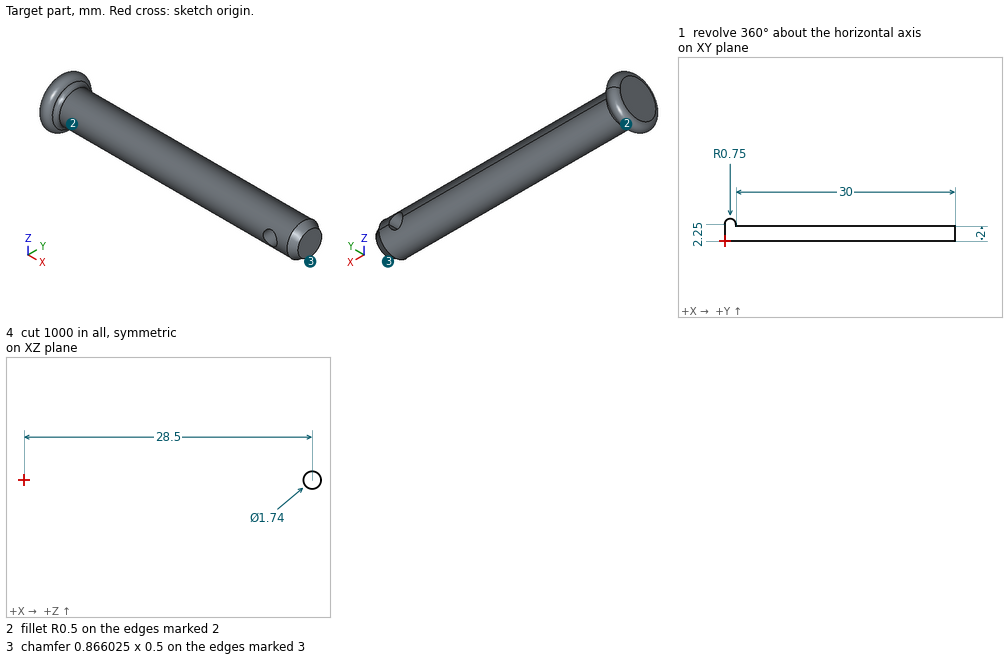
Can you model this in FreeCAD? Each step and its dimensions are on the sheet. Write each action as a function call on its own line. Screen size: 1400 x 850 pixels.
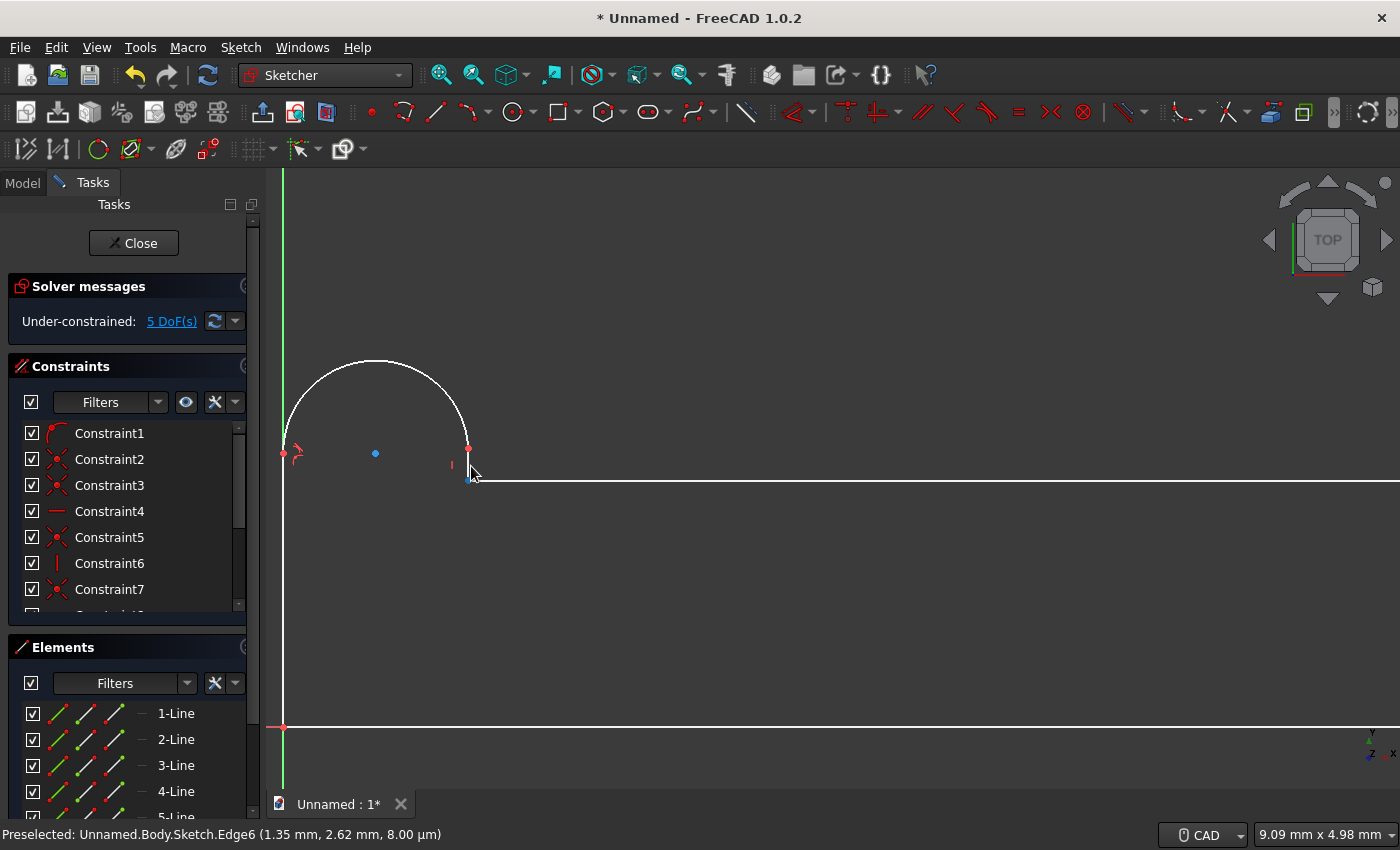
click(468, 465)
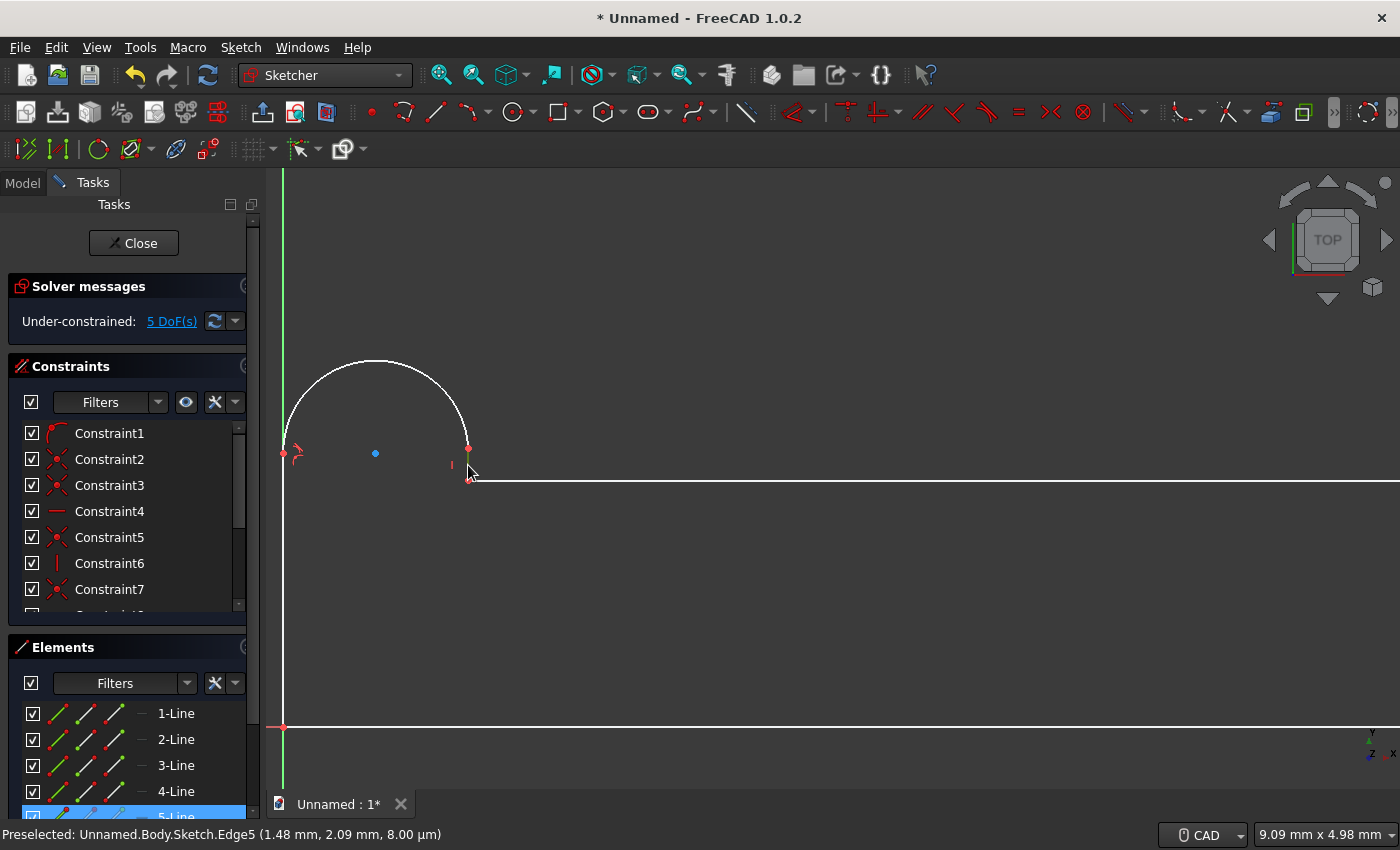
scroll(471, 466, down, 9)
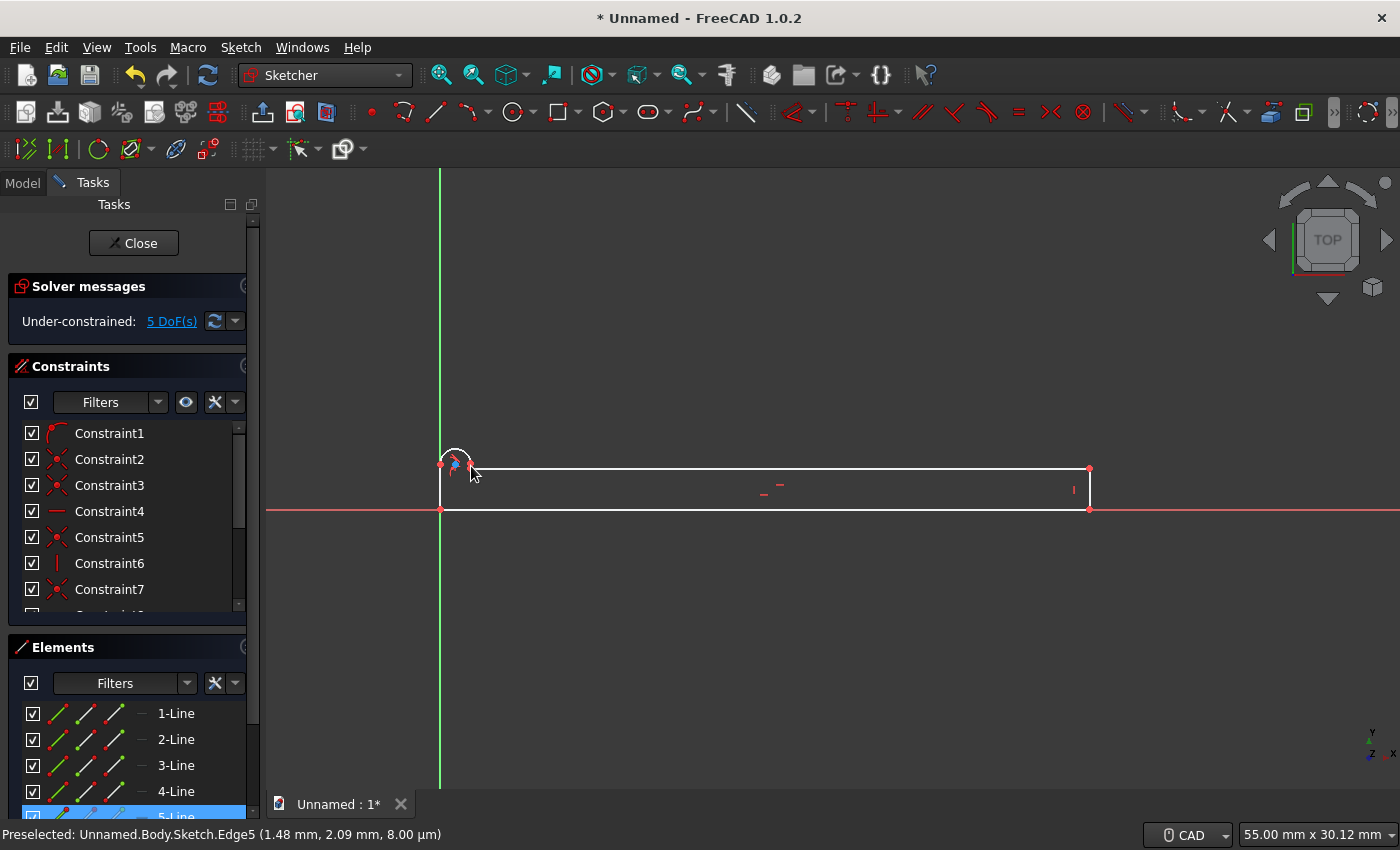
click(464, 452)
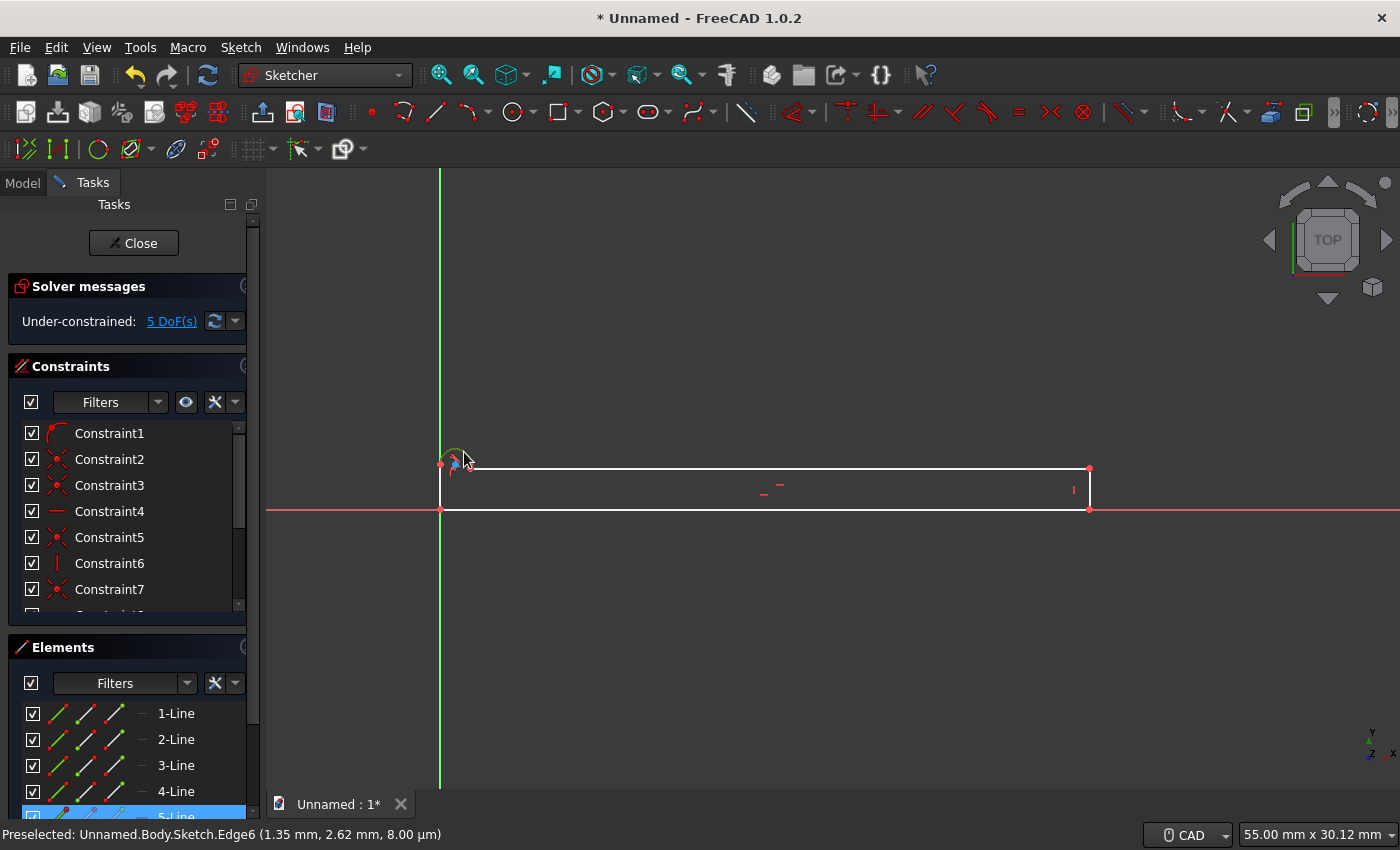
click(988, 112)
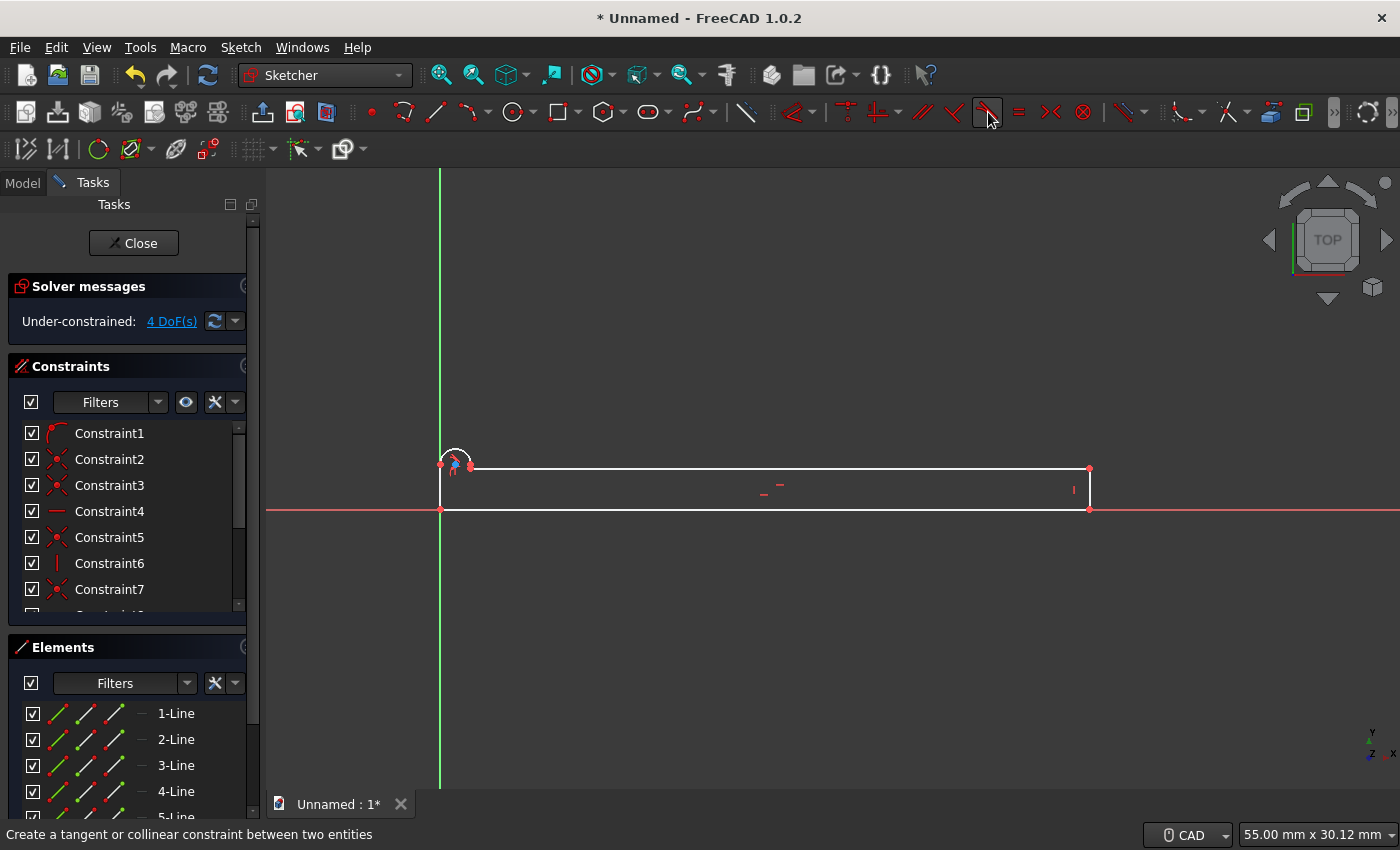
key(d)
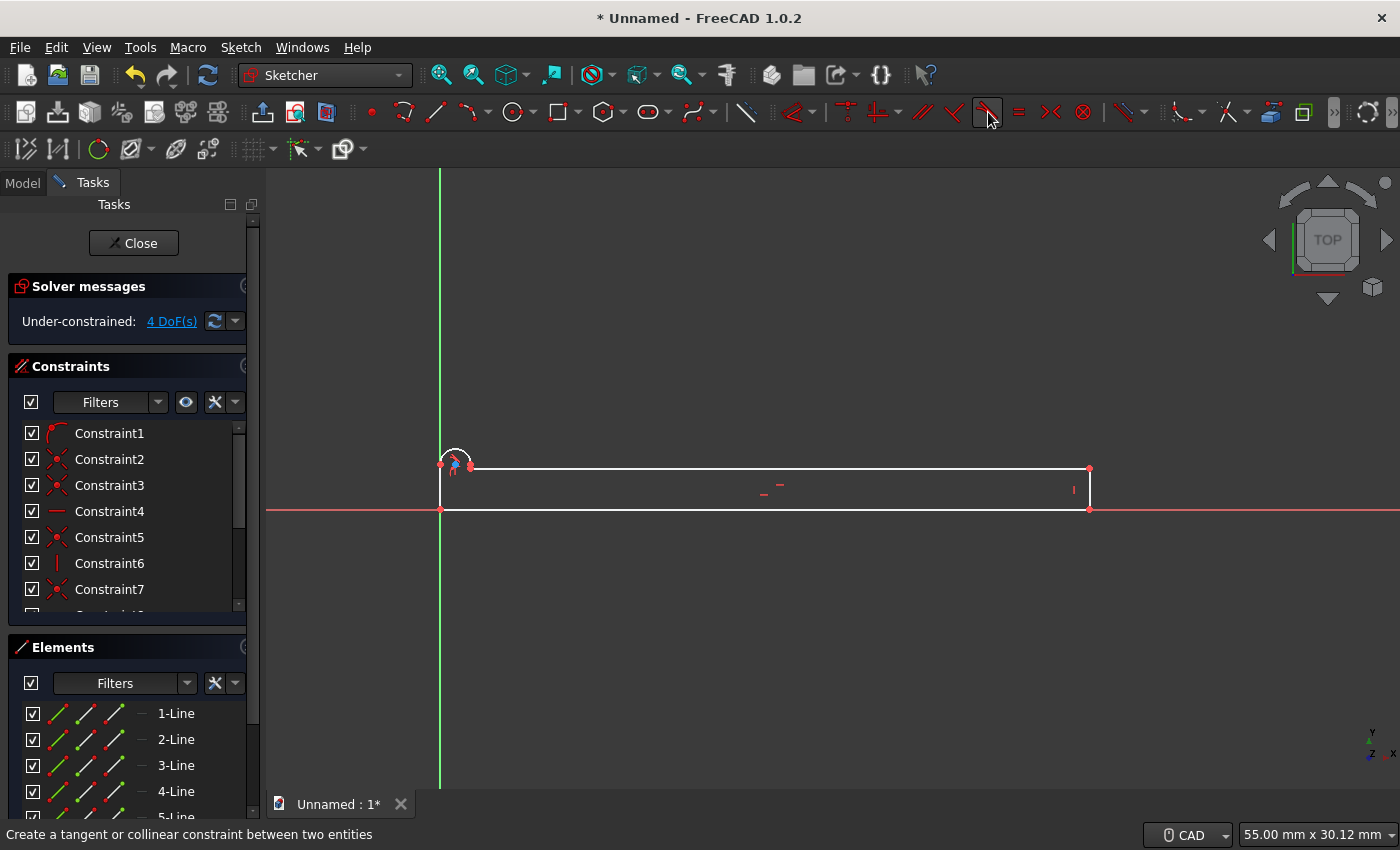
scroll(464, 452, up, 5)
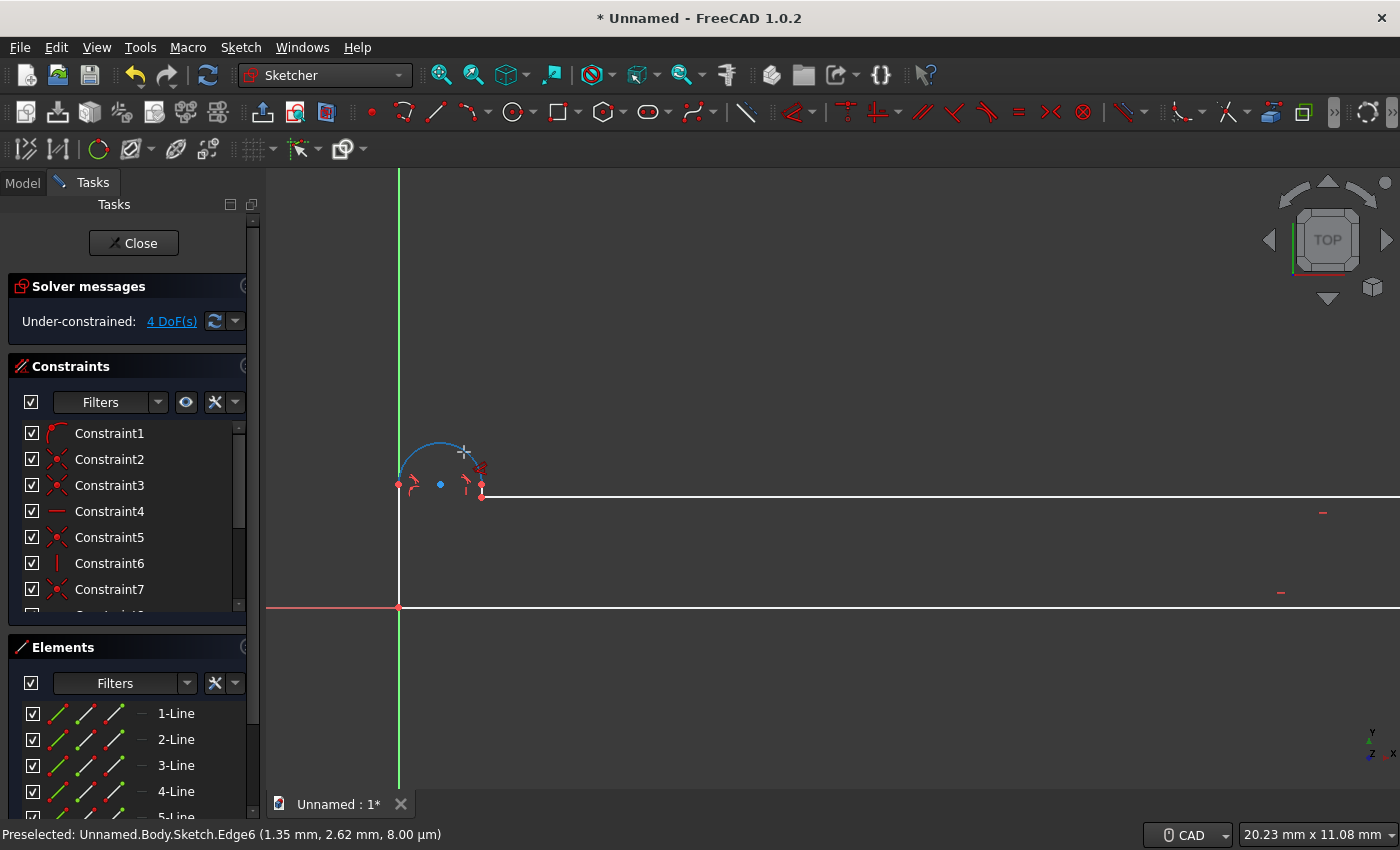
click(465, 451)
click(484, 425)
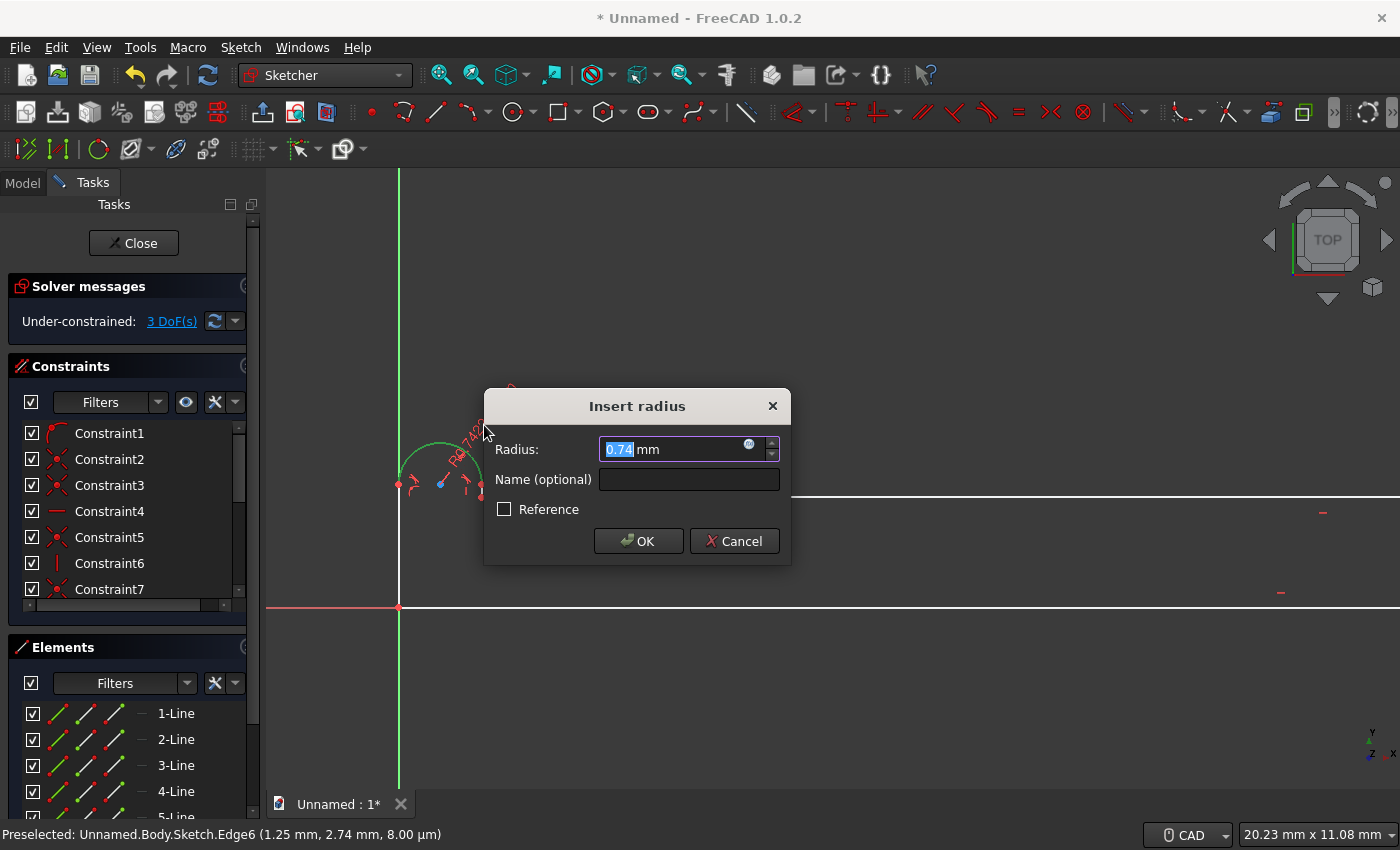
text(0.75)
key(Return)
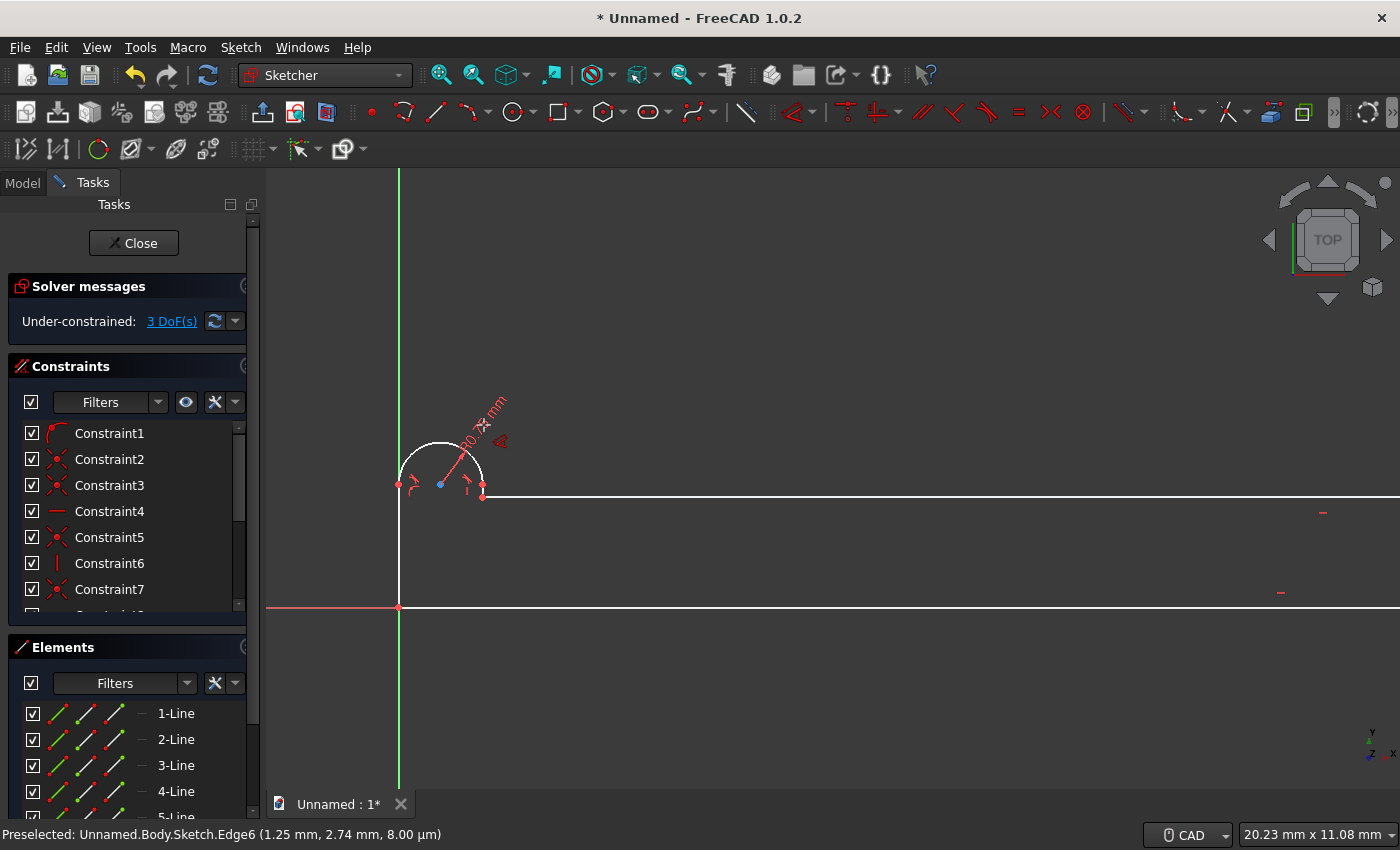
scroll(464, 452, down, 5)